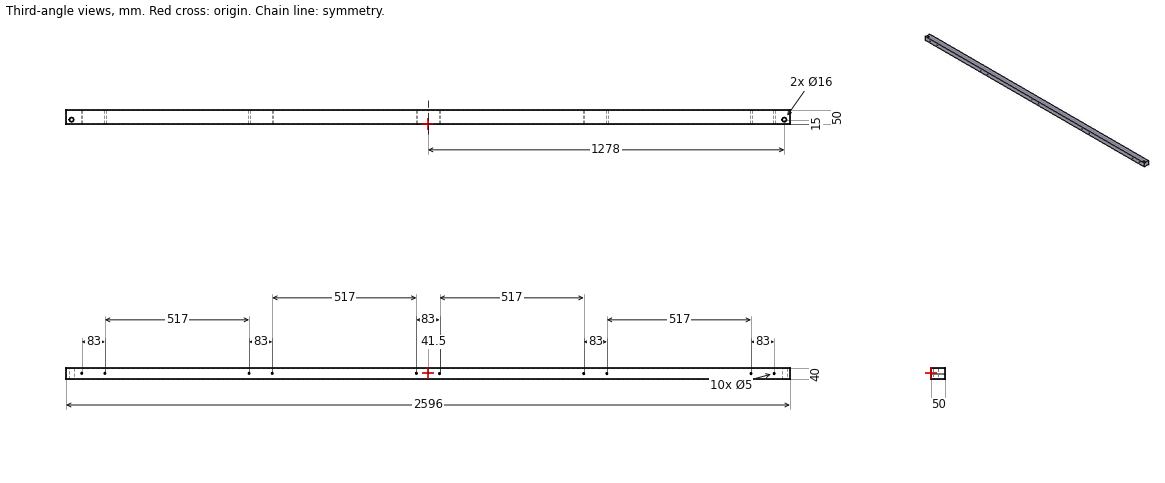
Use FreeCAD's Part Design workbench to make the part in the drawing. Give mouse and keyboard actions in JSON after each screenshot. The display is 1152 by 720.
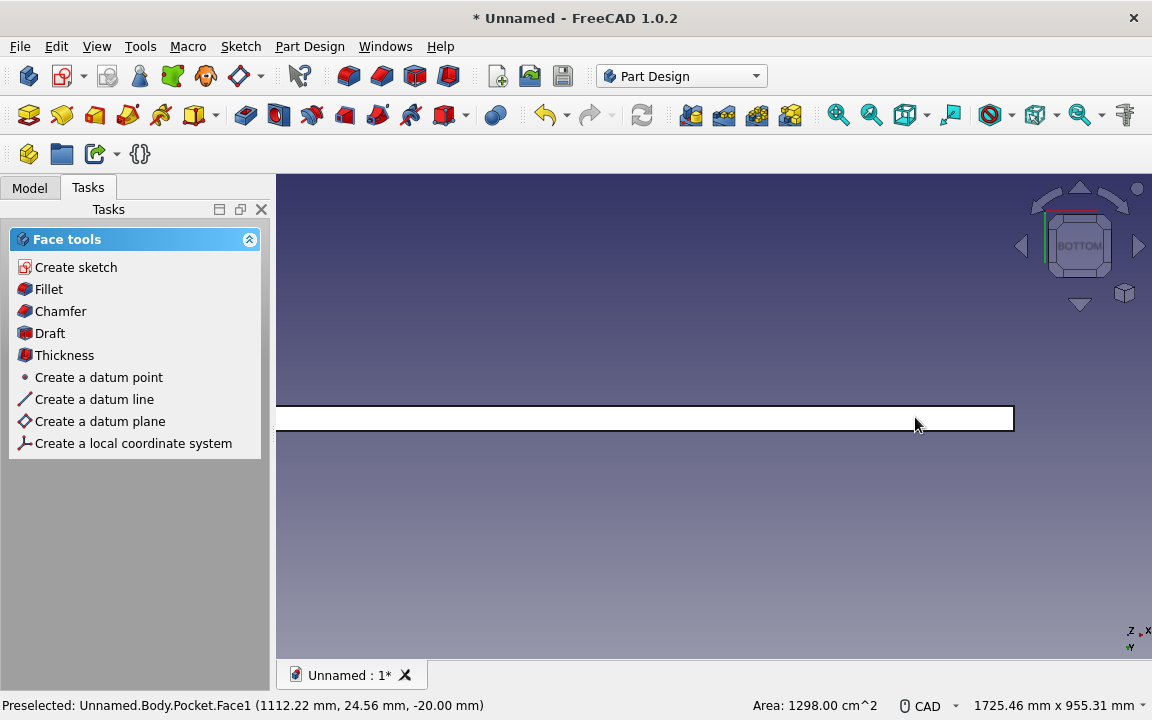
{"action": "left_click", "coordinate": [62, 76]}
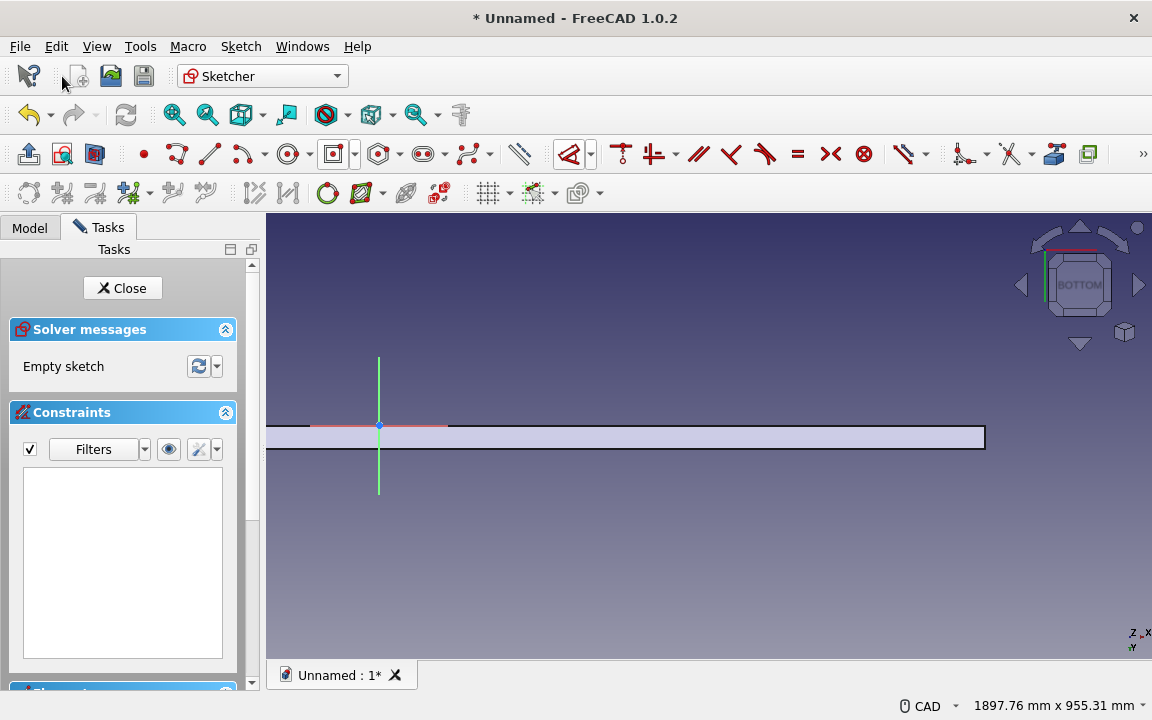
{"action": "scroll", "coordinate": [854, 440], "scroll_direction": "down", "scroll_amount": 4}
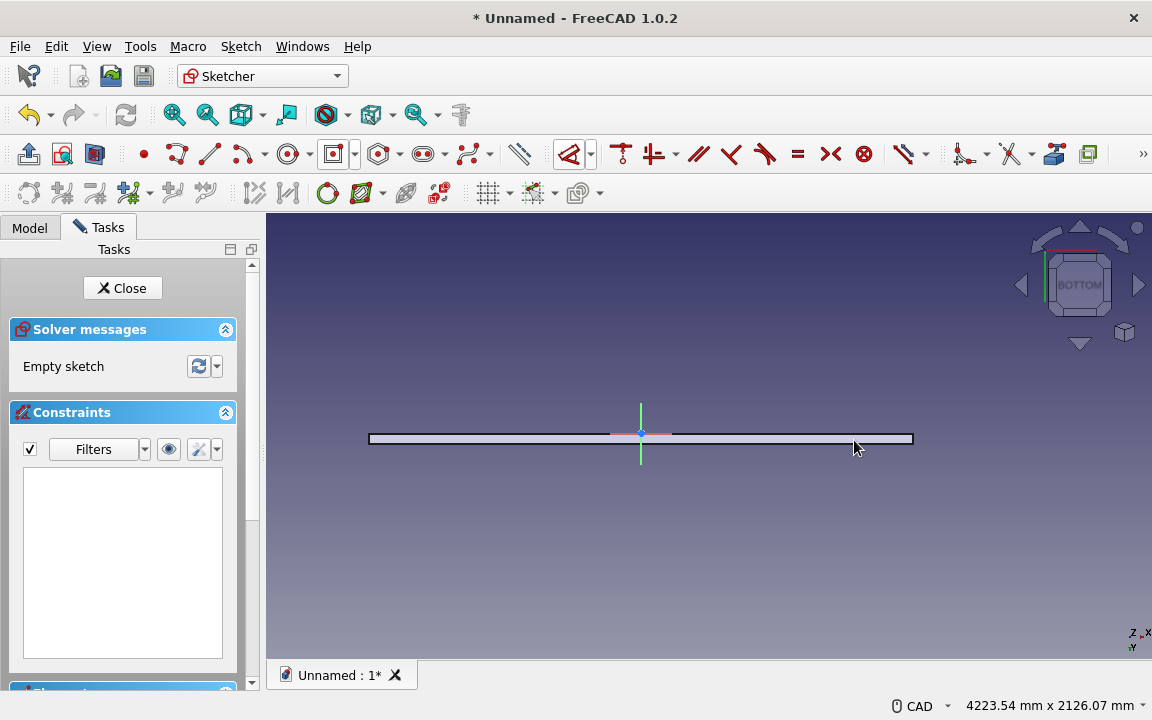
{"action": "left_click", "coordinate": [288, 154]}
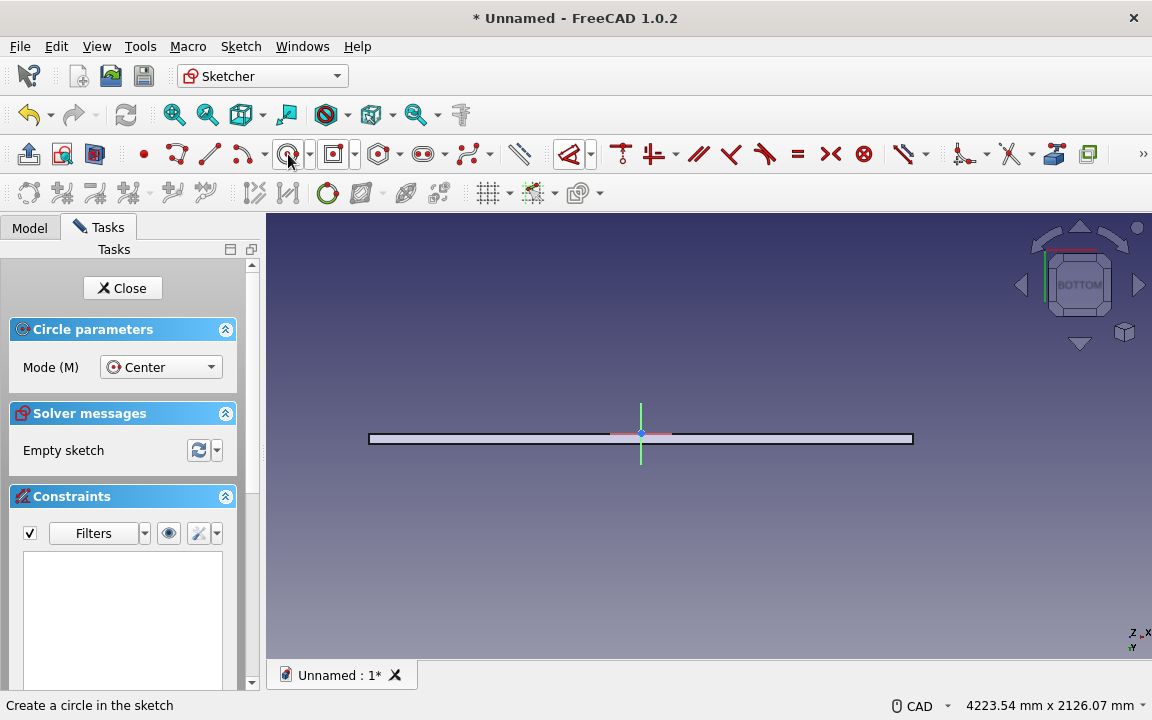
{"action": "scroll", "coordinate": [909, 437], "scroll_direction": "up", "scroll_amount": 14}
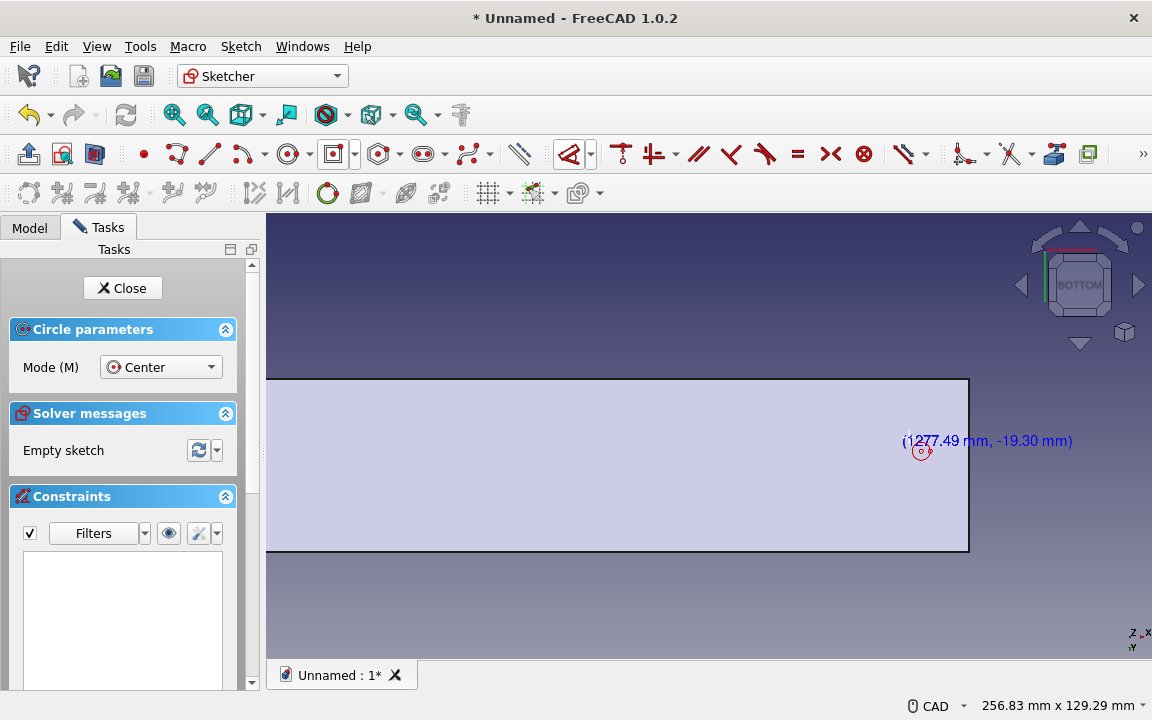
{"action": "scroll", "coordinate": [909, 437], "scroll_direction": "down", "scroll_amount": 14}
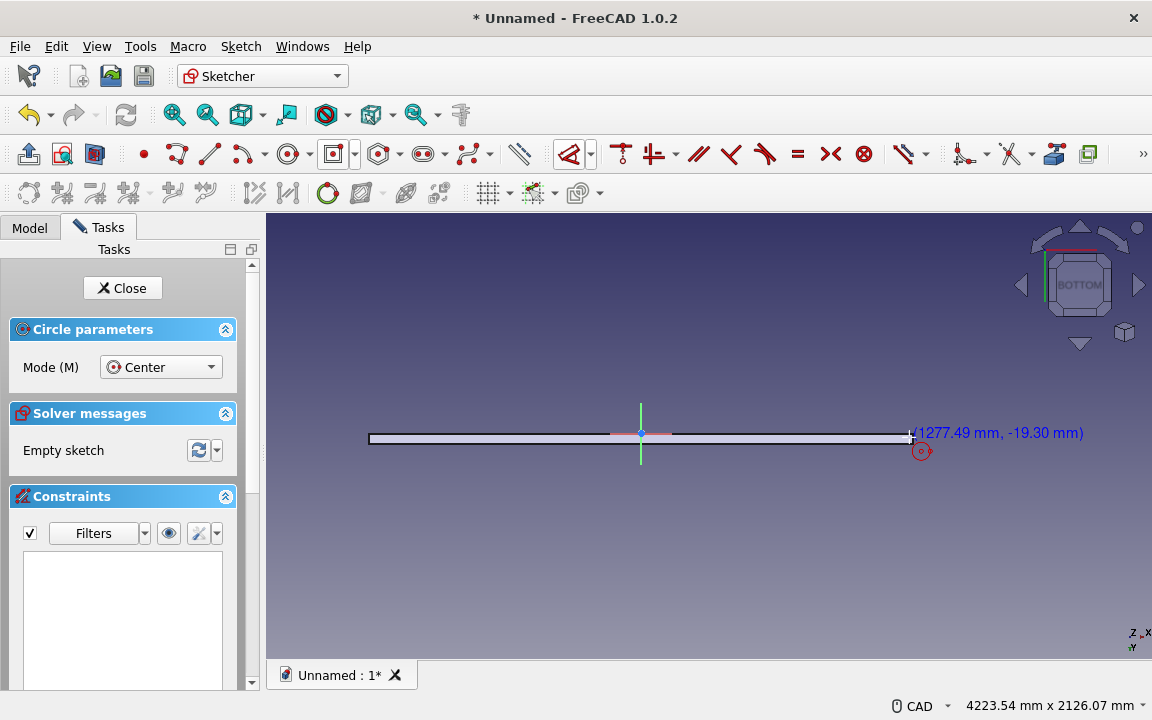
{"action": "scroll", "coordinate": [909, 437], "scroll_direction": "up", "scroll_amount": 9}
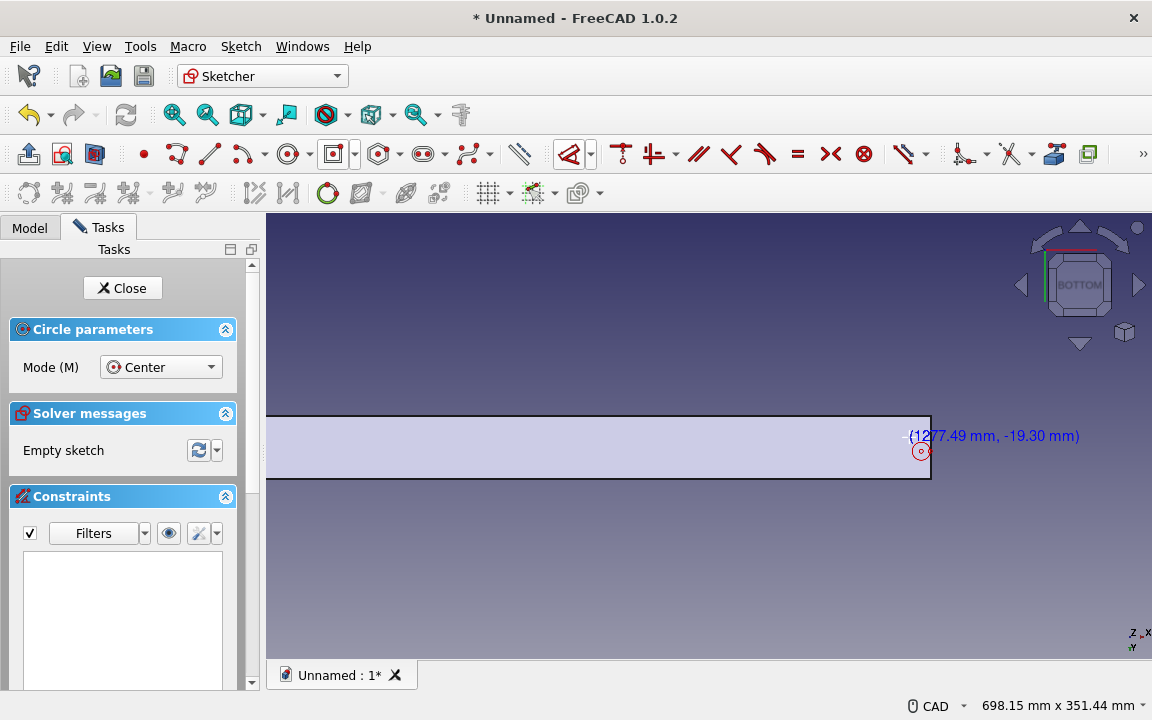
{"action": "left_click", "coordinate": [906, 435]}
{"action": "mouse_move", "coordinate": [913, 442]}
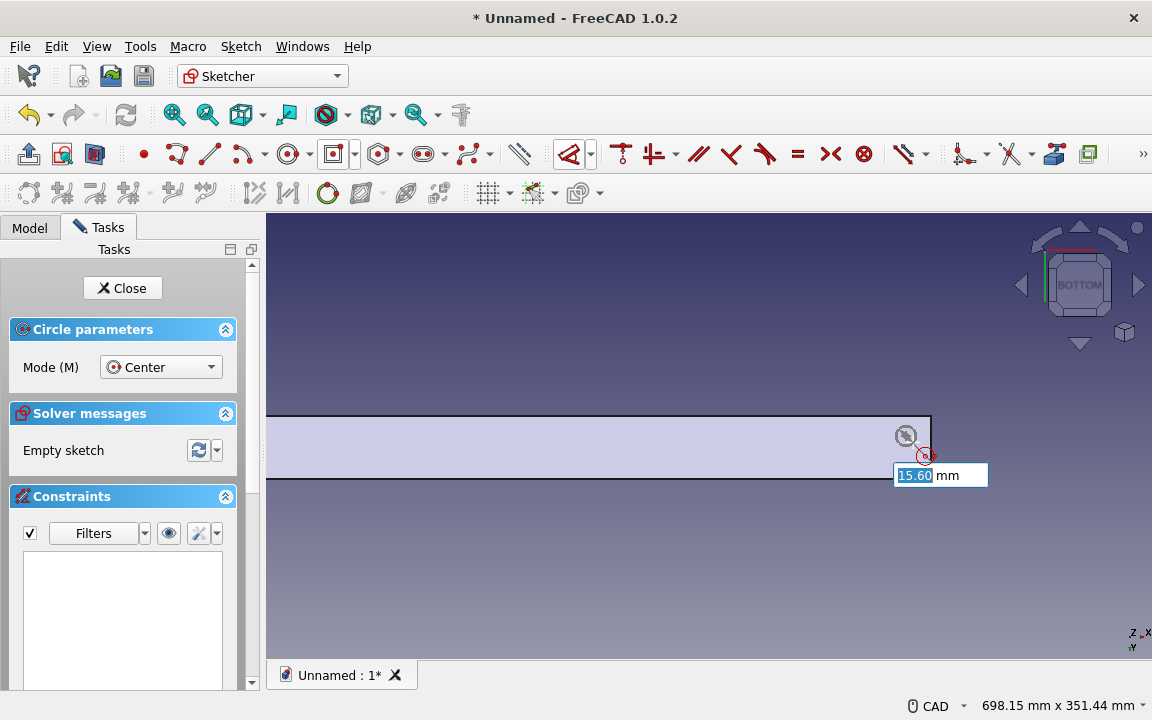
{"action": "type", "text": "16"}
{"action": "key", "text": "Return"}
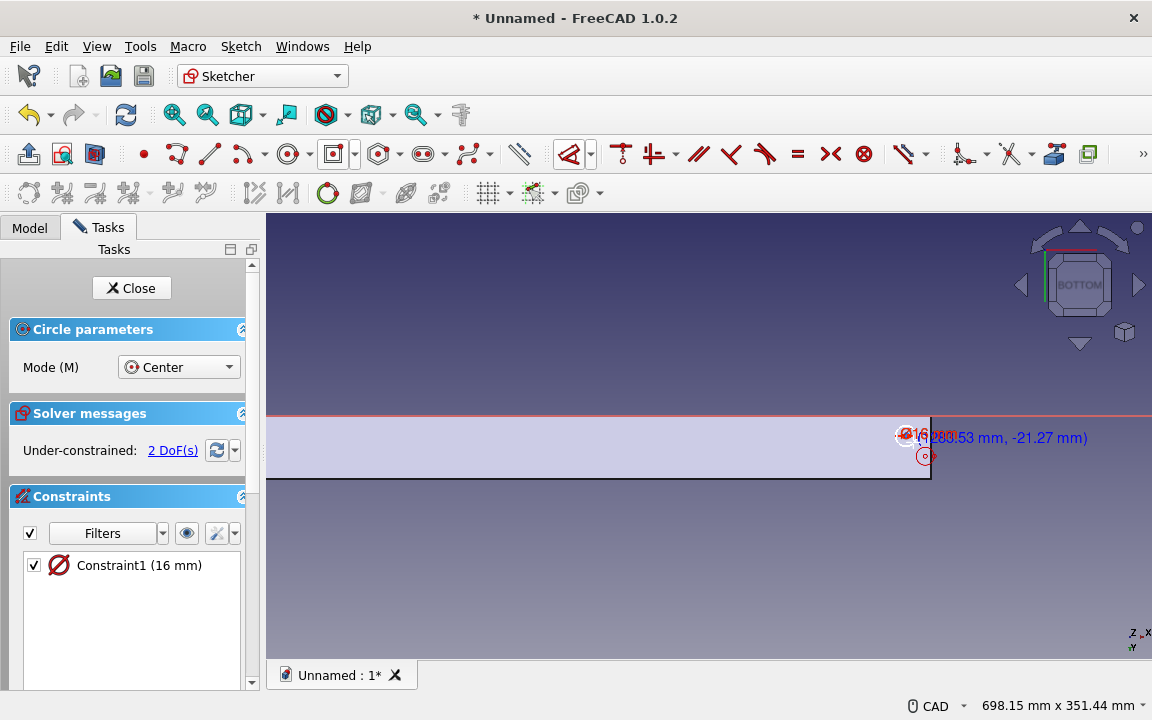
{"action": "scroll", "coordinate": [909, 437], "scroll_direction": "down", "scroll_amount": 9}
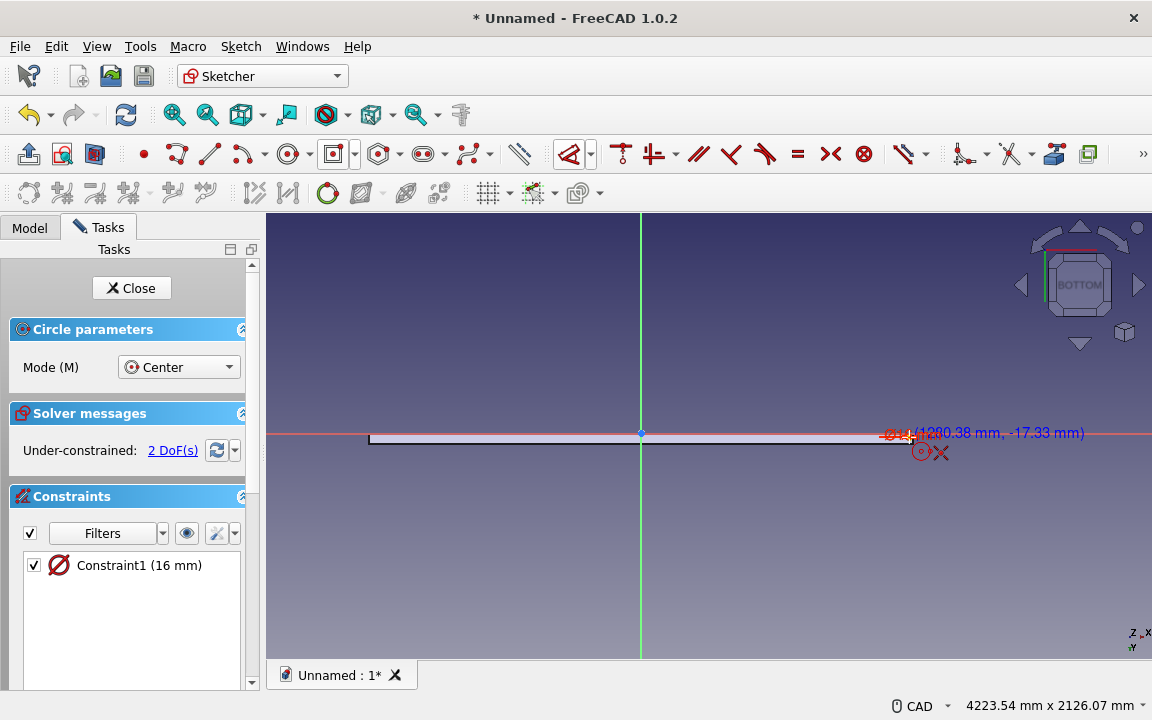
{"action": "scroll", "coordinate": [373, 437], "scroll_direction": "up", "scroll_amount": 14}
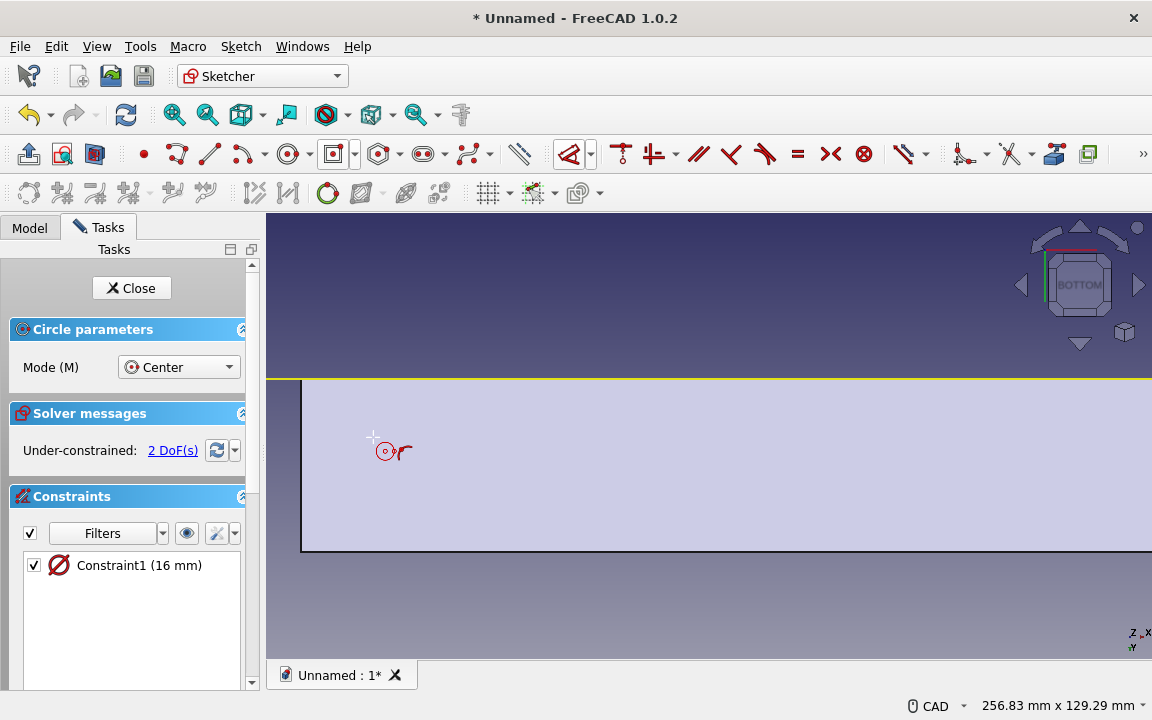
{"action": "scroll", "coordinate": [373, 437], "scroll_direction": "down", "scroll_amount": 14}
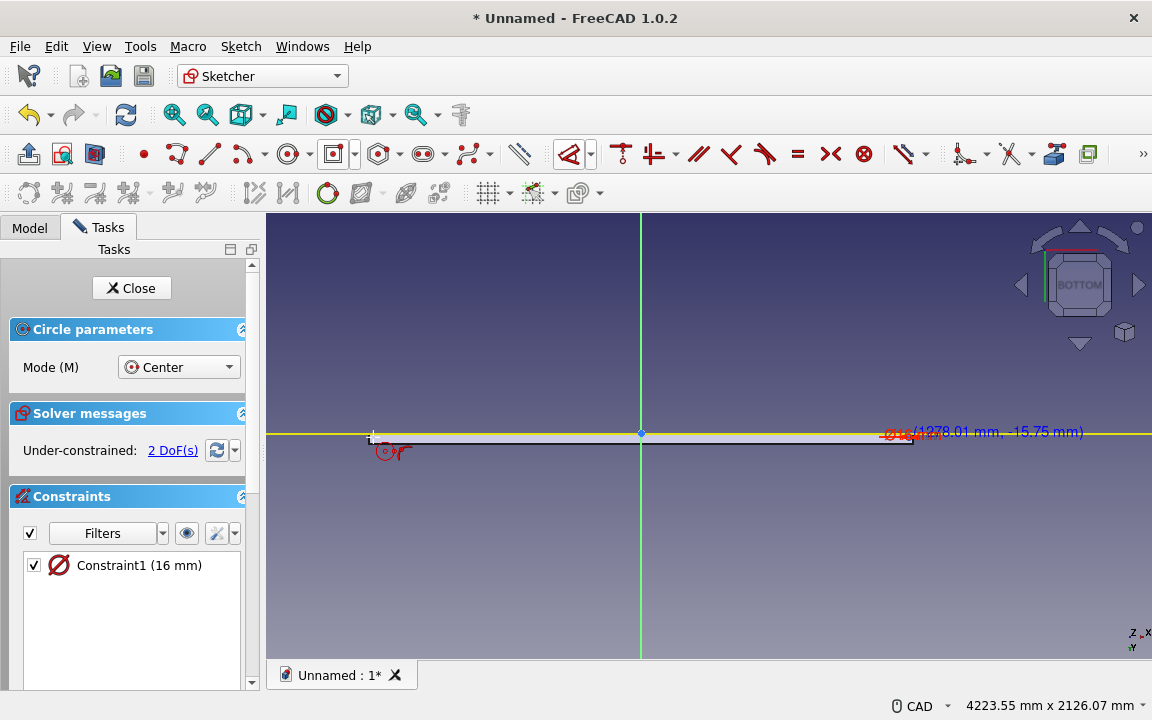
{"action": "scroll", "coordinate": [373, 437], "scroll_direction": "up", "scroll_amount": 9}